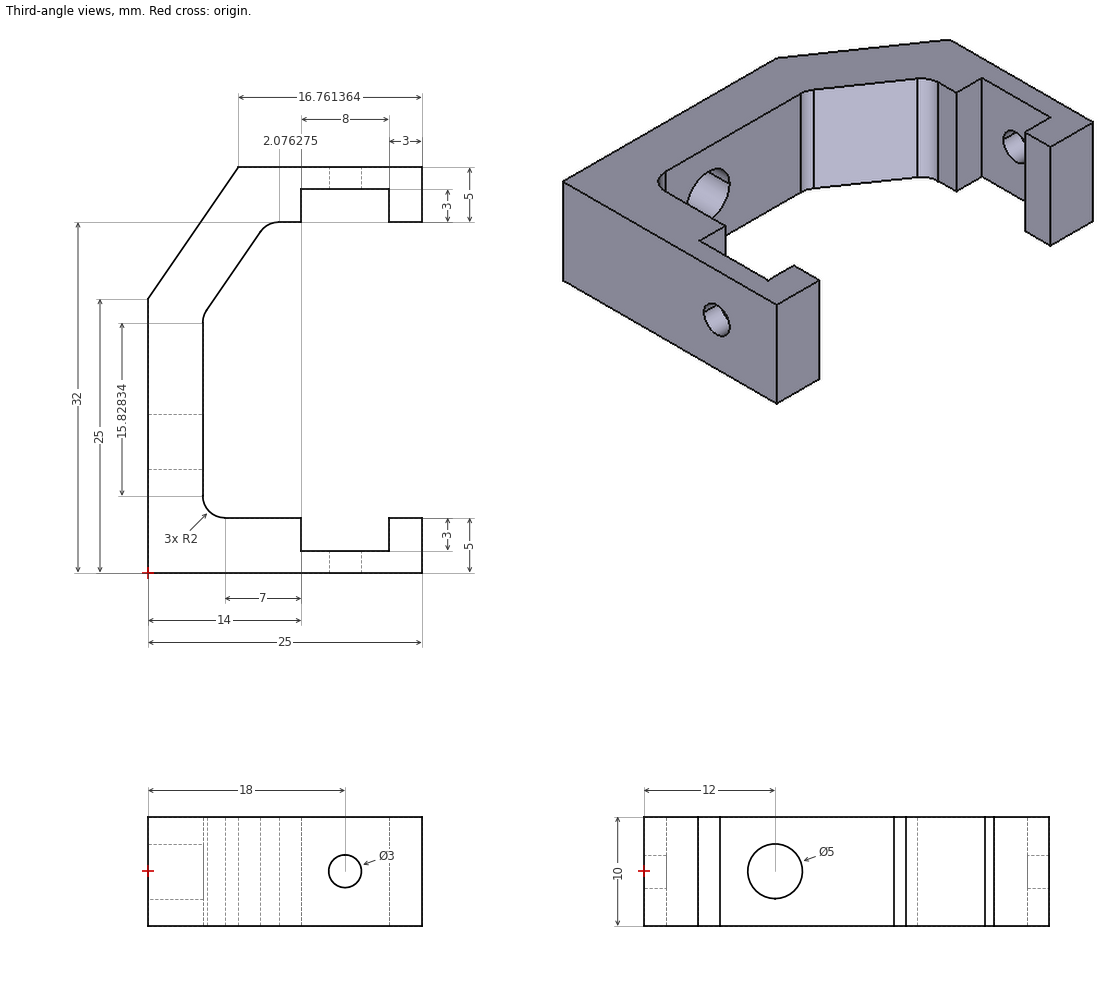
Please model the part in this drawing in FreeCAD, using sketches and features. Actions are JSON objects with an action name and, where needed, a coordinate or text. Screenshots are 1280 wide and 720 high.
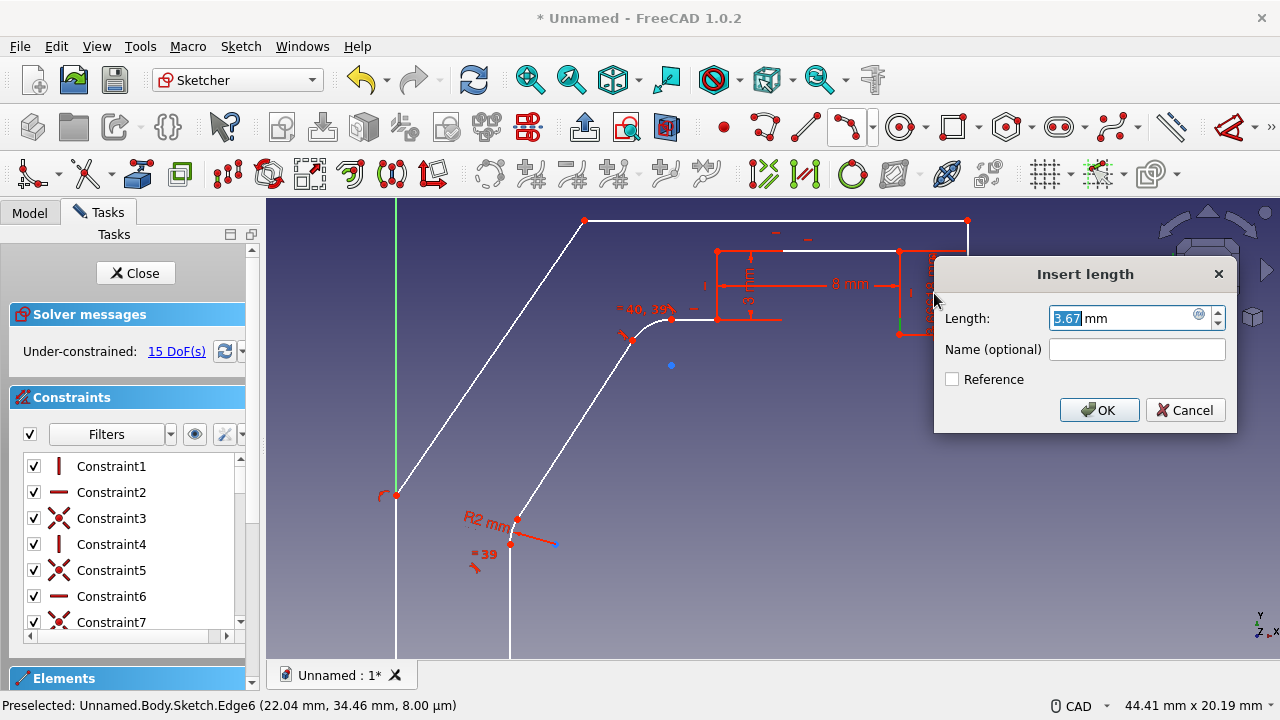
{"action": "type", "text": "3"}
{"action": "key", "text": "Return"}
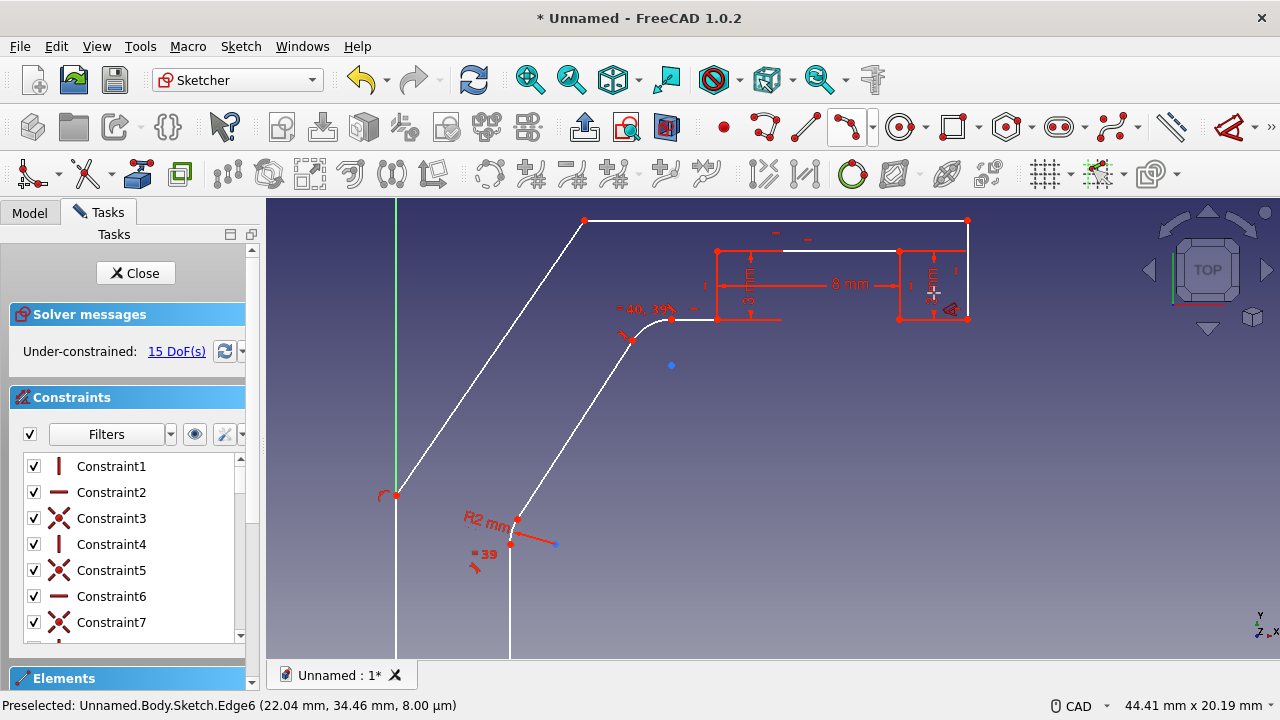
{"action": "left_click", "coordinate": [920, 320]}
{"action": "left_click", "coordinate": [934, 354]}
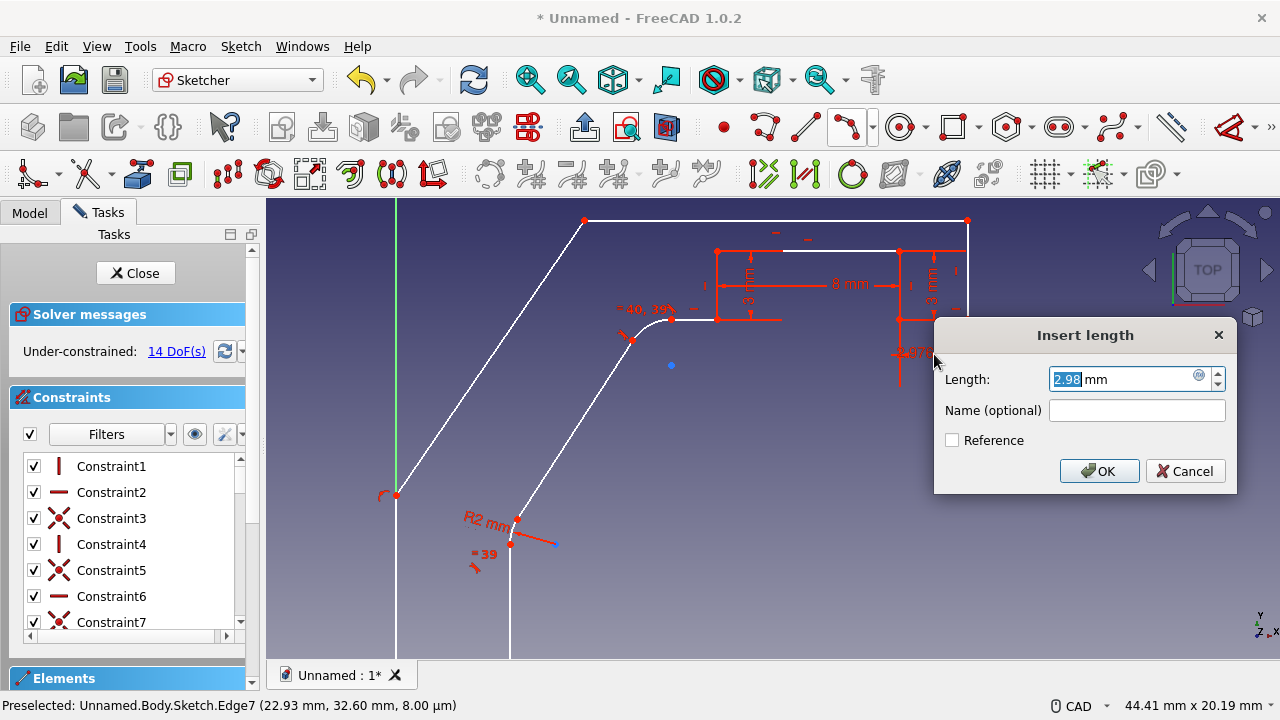
{"action": "type", "text": "3"}
{"action": "key", "text": "Return"}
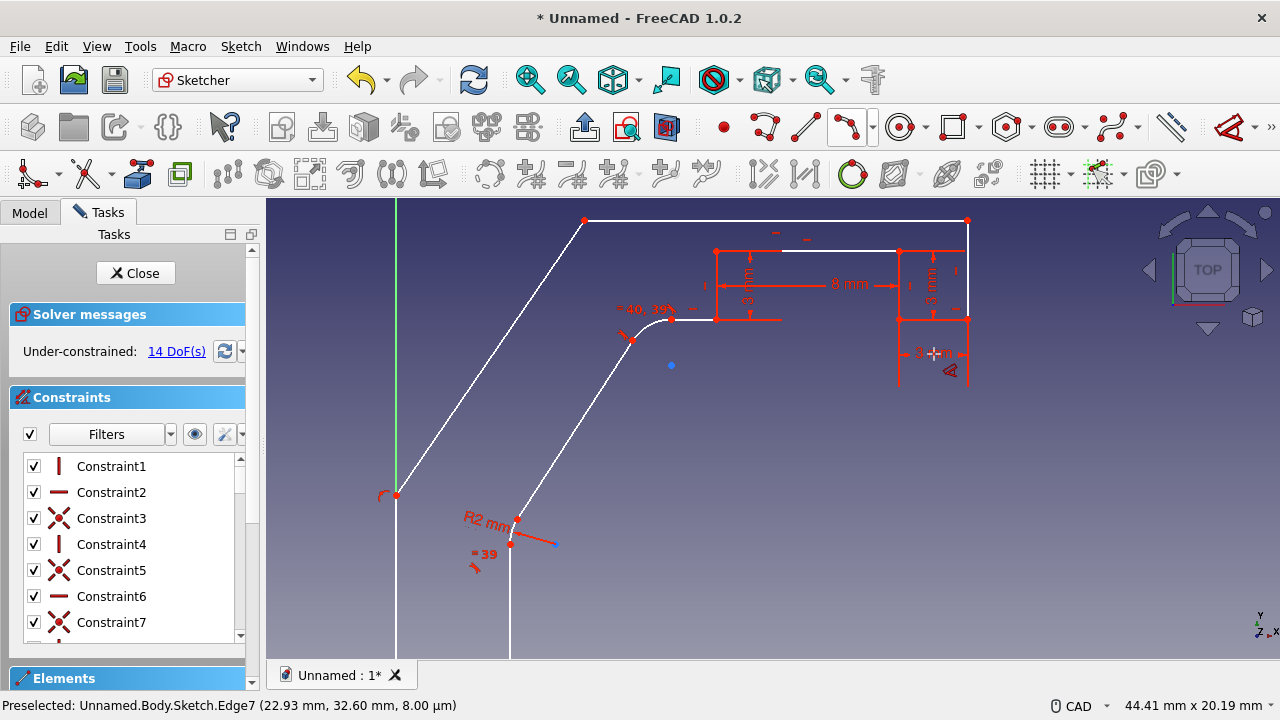
{"action": "left_click", "coordinate": [968, 290]}
{"action": "left_click", "coordinate": [1002, 273]}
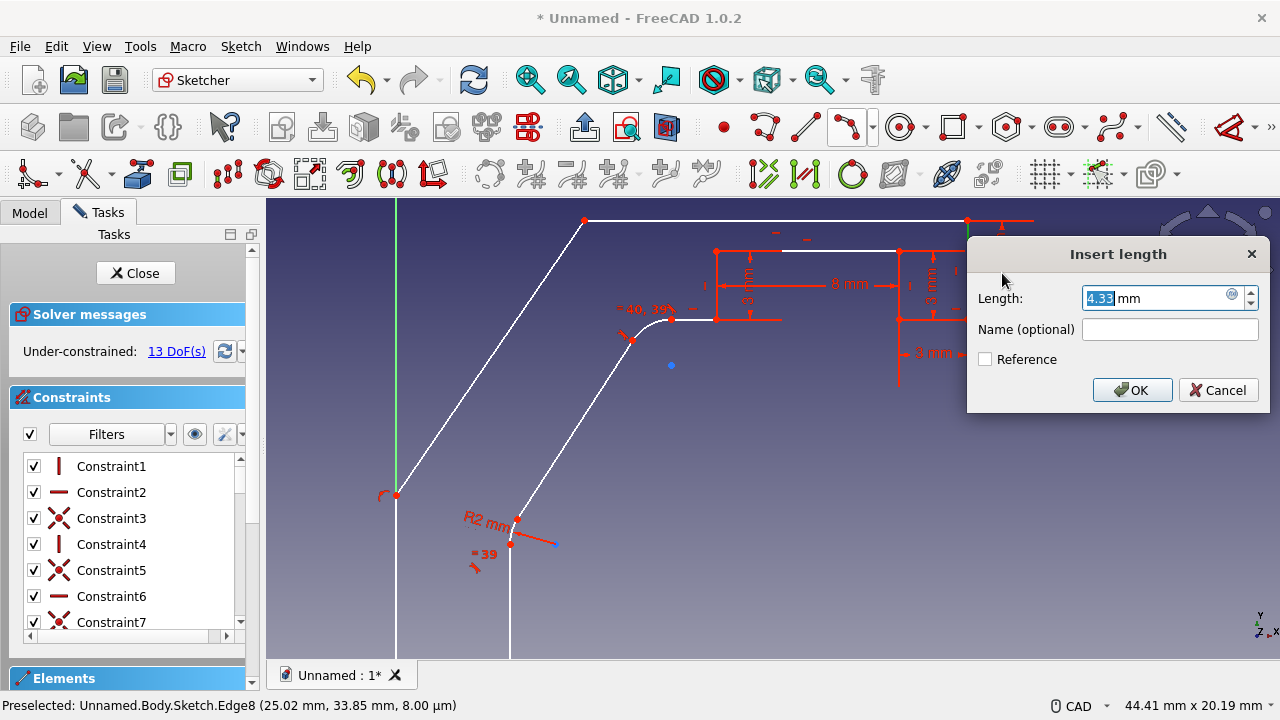
{"action": "type", "text": "5"}
{"action": "key", "text": "Return"}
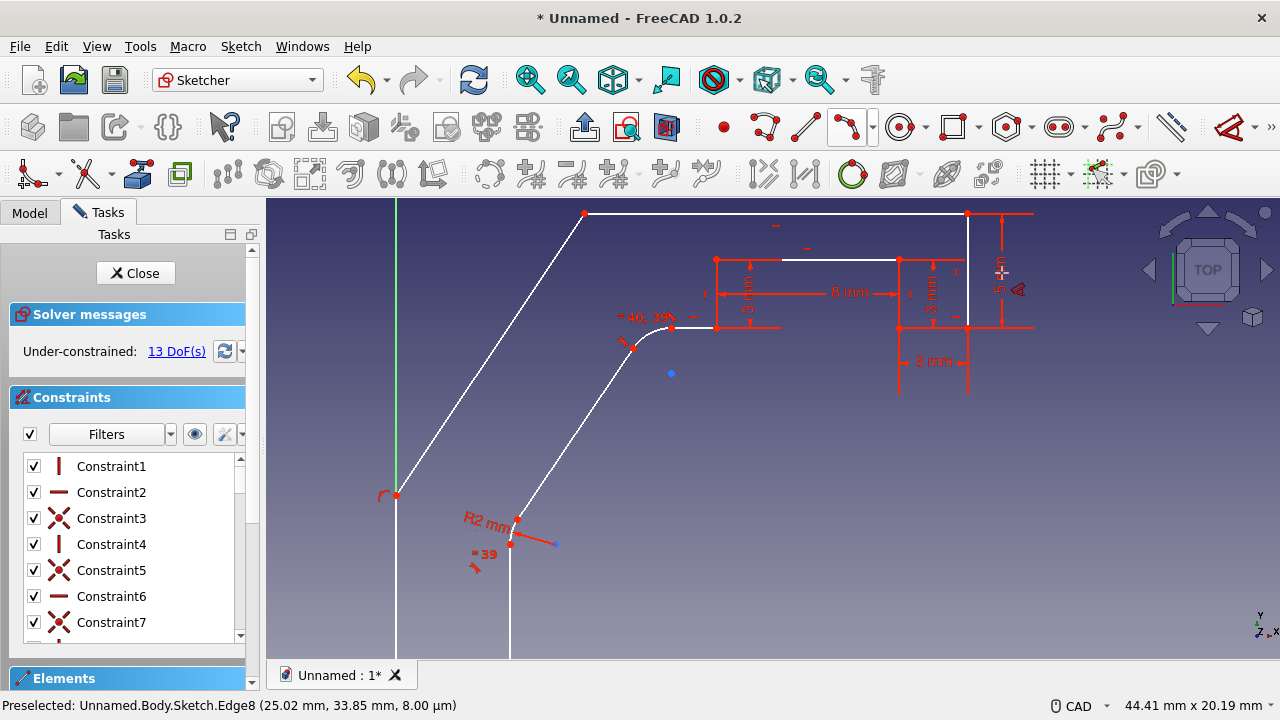
{"action": "scroll", "coordinate": [718, 305], "scroll_direction": "down", "scroll_amount": 5}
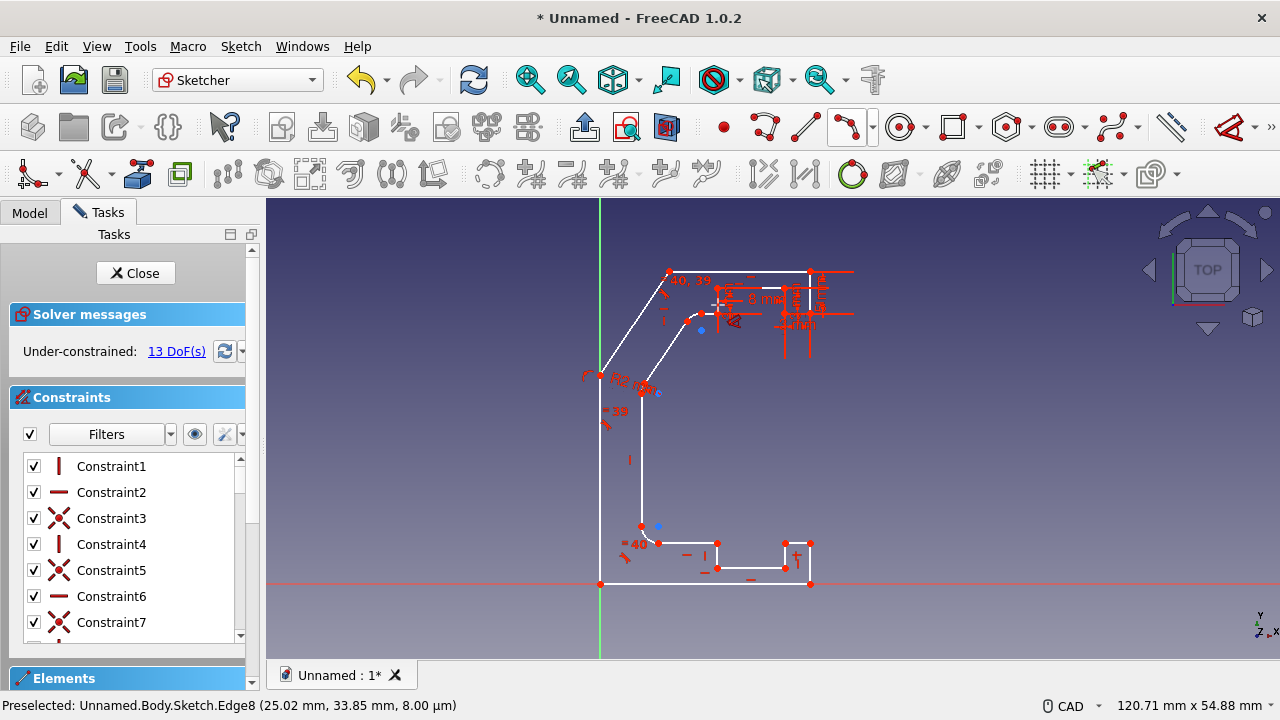
{"action": "left_click", "coordinate": [810, 572]}
{"action": "left_click", "coordinate": [844, 564]}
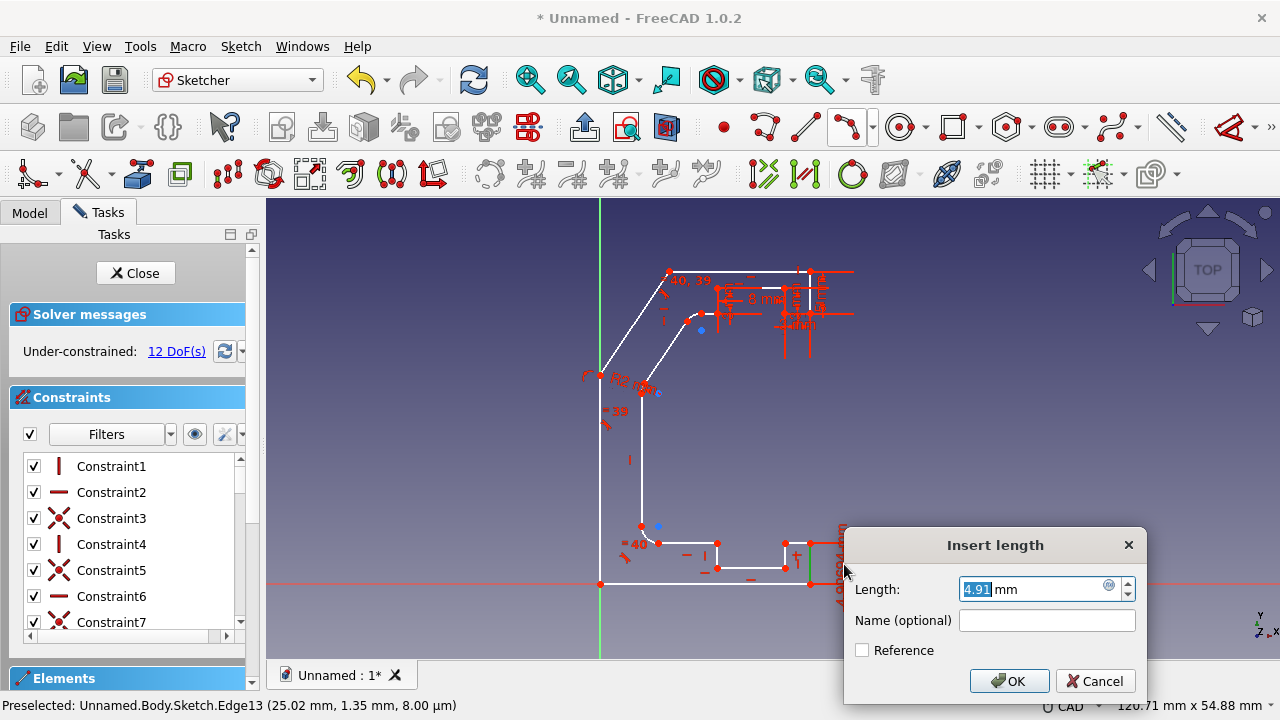
{"action": "type", "text": "5"}
{"action": "key", "text": "Return"}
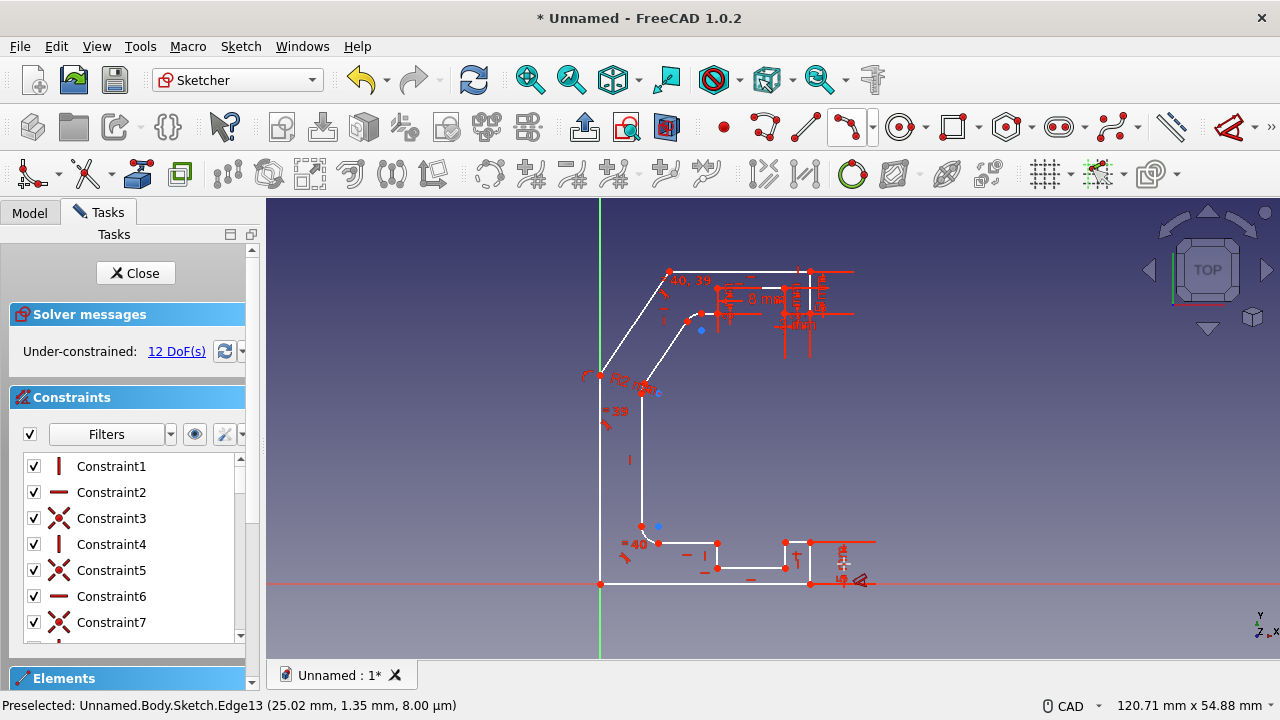
{"action": "scroll", "coordinate": [800, 542], "scroll_direction": "up", "scroll_amount": 3}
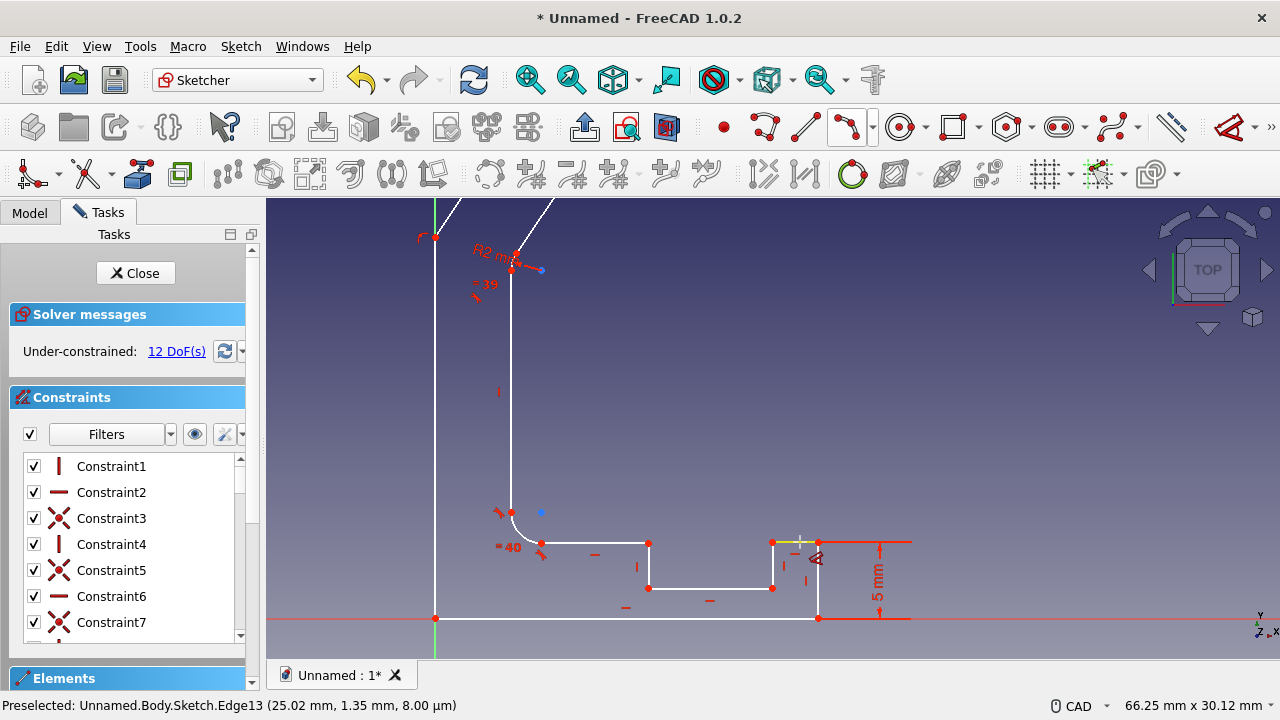
{"action": "left_click", "coordinate": [800, 542]}
{"action": "left_click", "coordinate": [795, 576]}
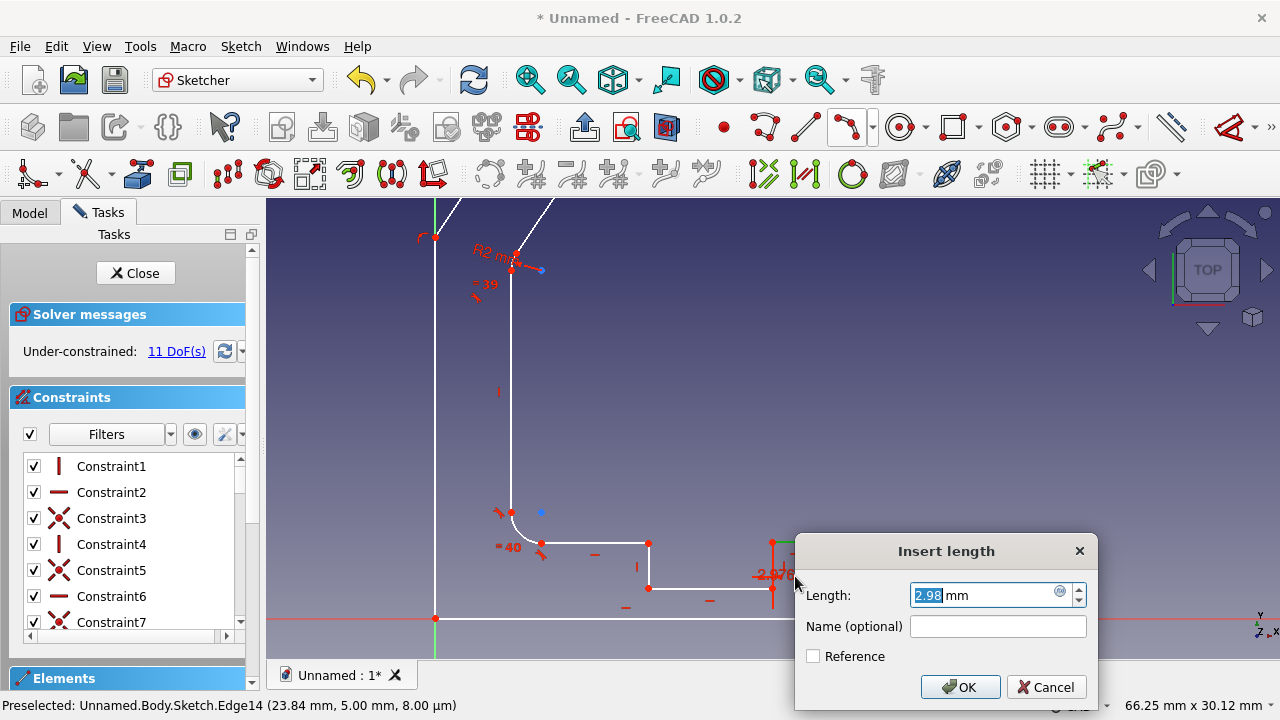
{"action": "type", "text": "3"}
{"action": "key", "text": "Return"}